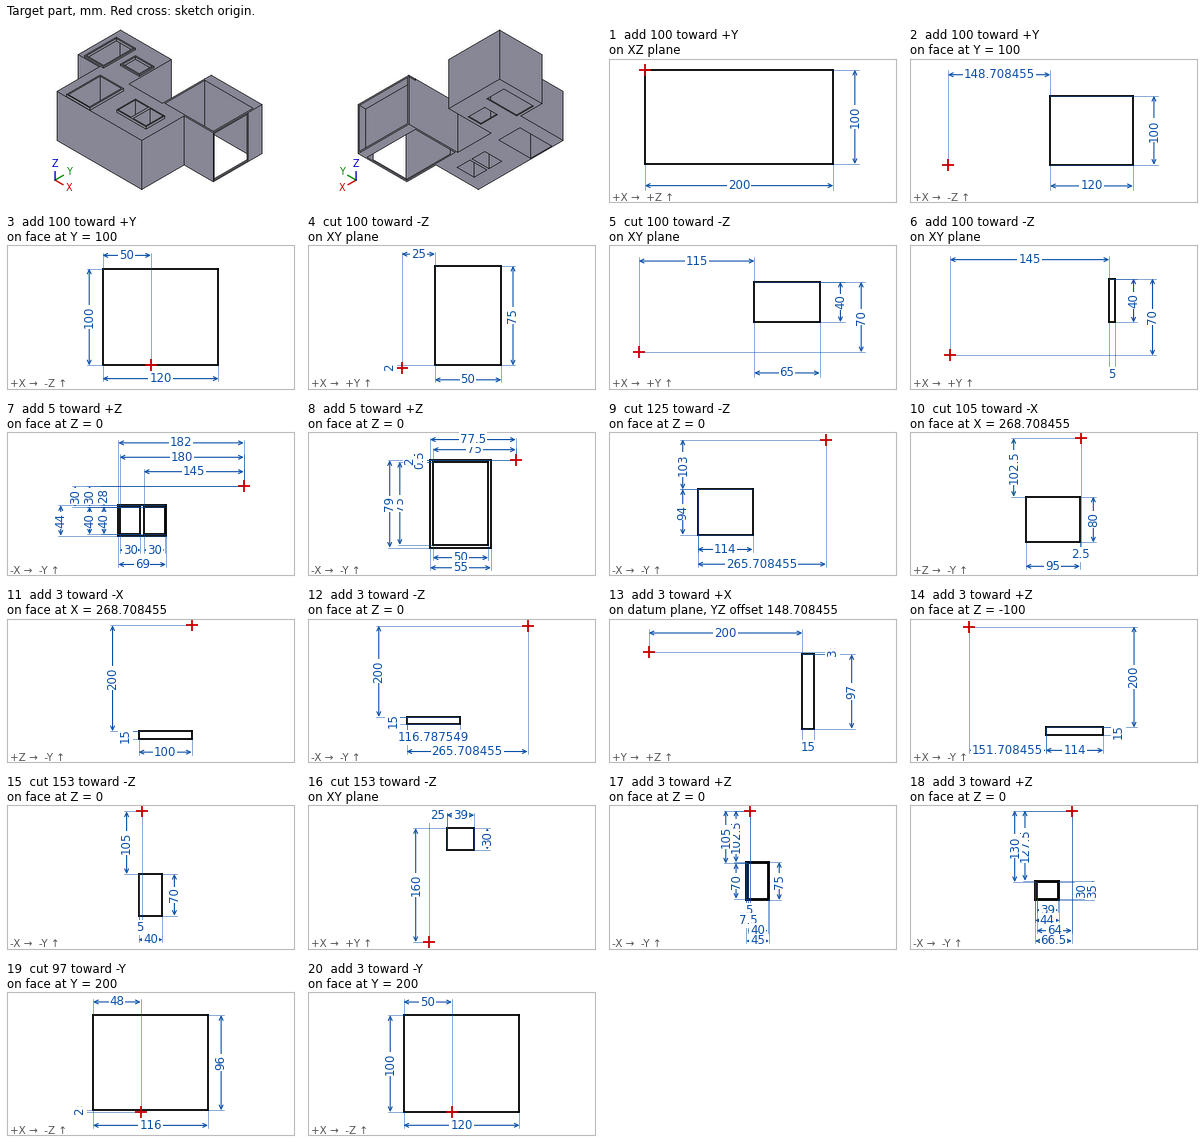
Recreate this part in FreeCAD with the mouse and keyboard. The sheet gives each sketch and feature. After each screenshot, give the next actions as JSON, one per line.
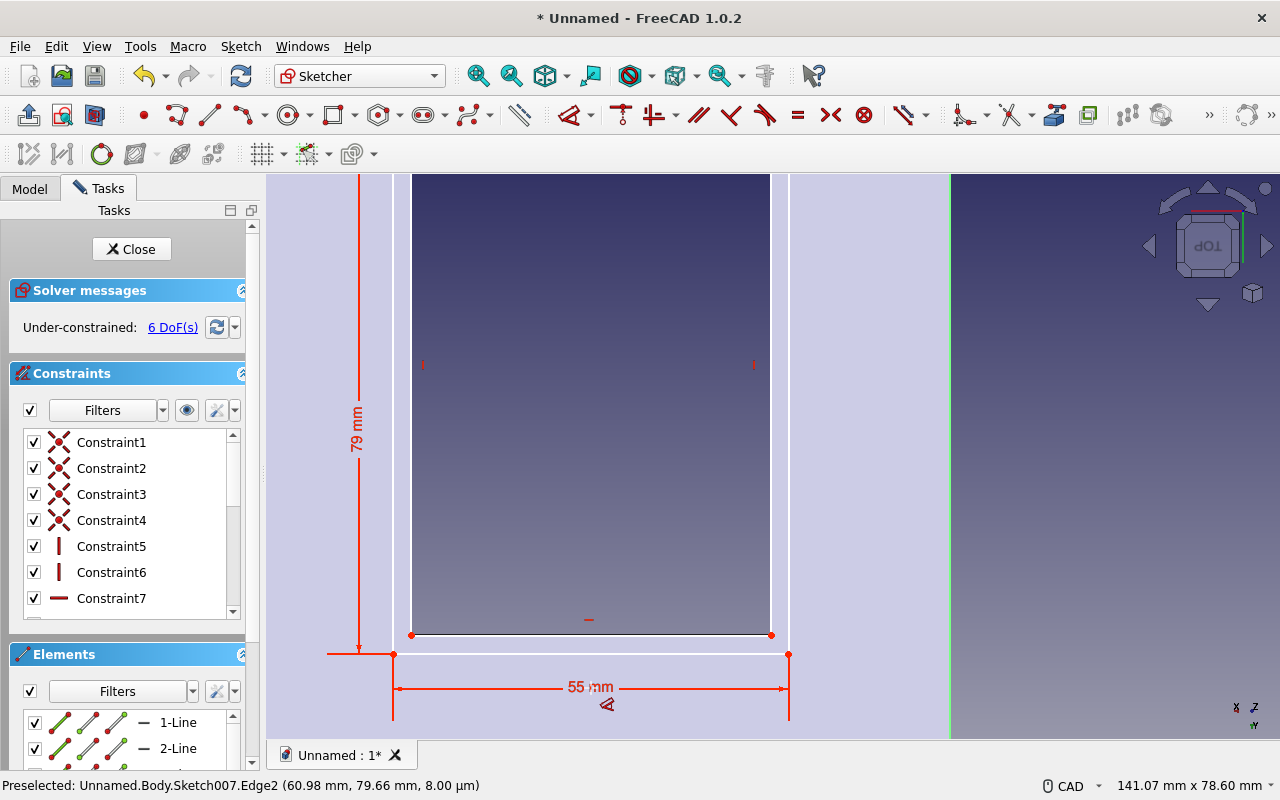
{"action": "left_click", "coordinate": [411, 259]}
{"action": "left_click", "coordinate": [377, 319]}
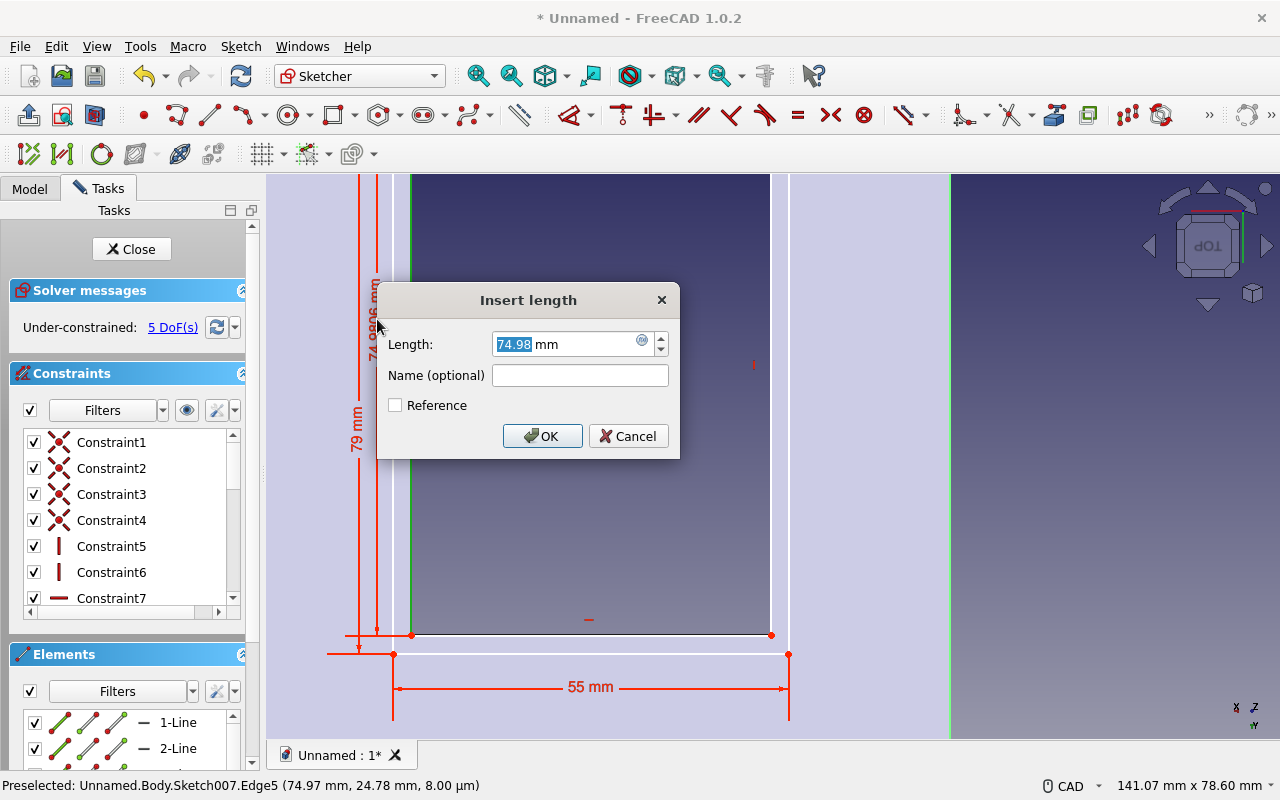
{"action": "type", "text": "75"}
{"action": "key", "text": "Return"}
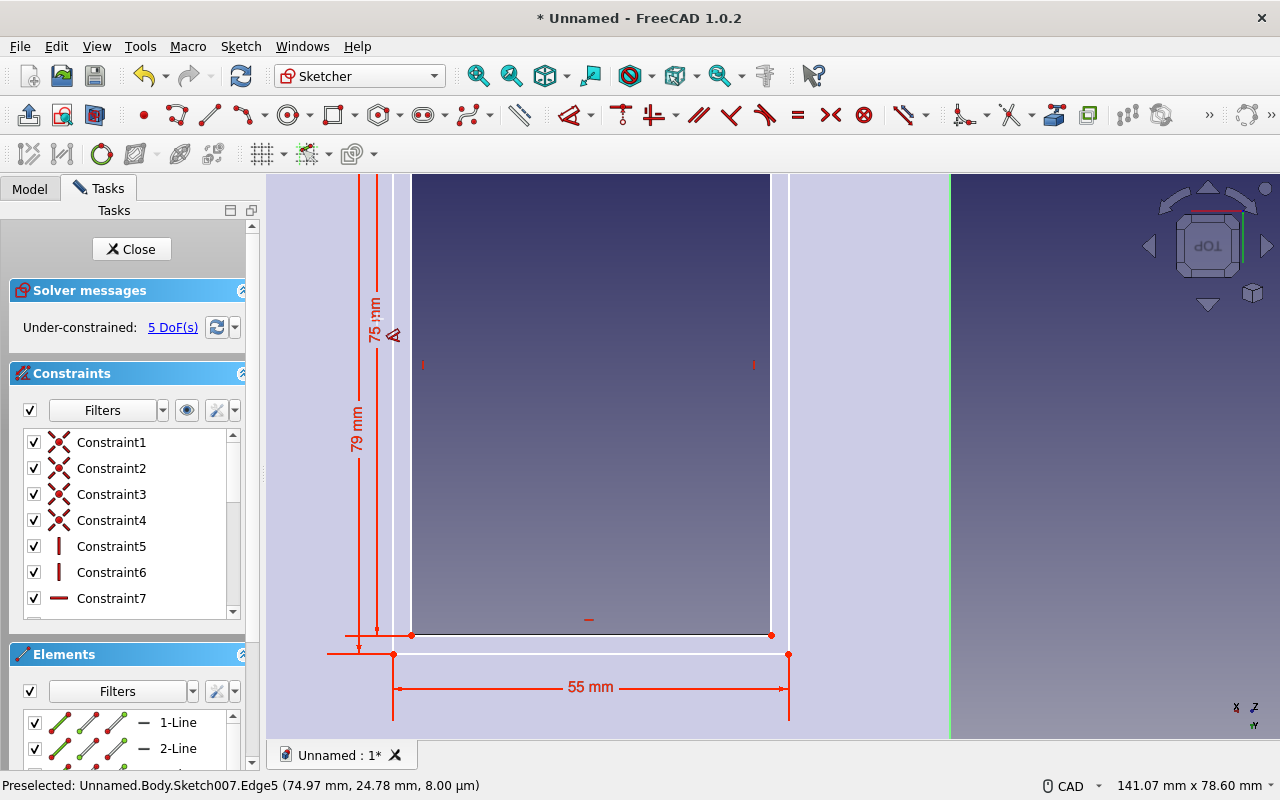
{"action": "left_click", "coordinate": [519, 636]}
{"action": "left_click", "coordinate": [509, 670]}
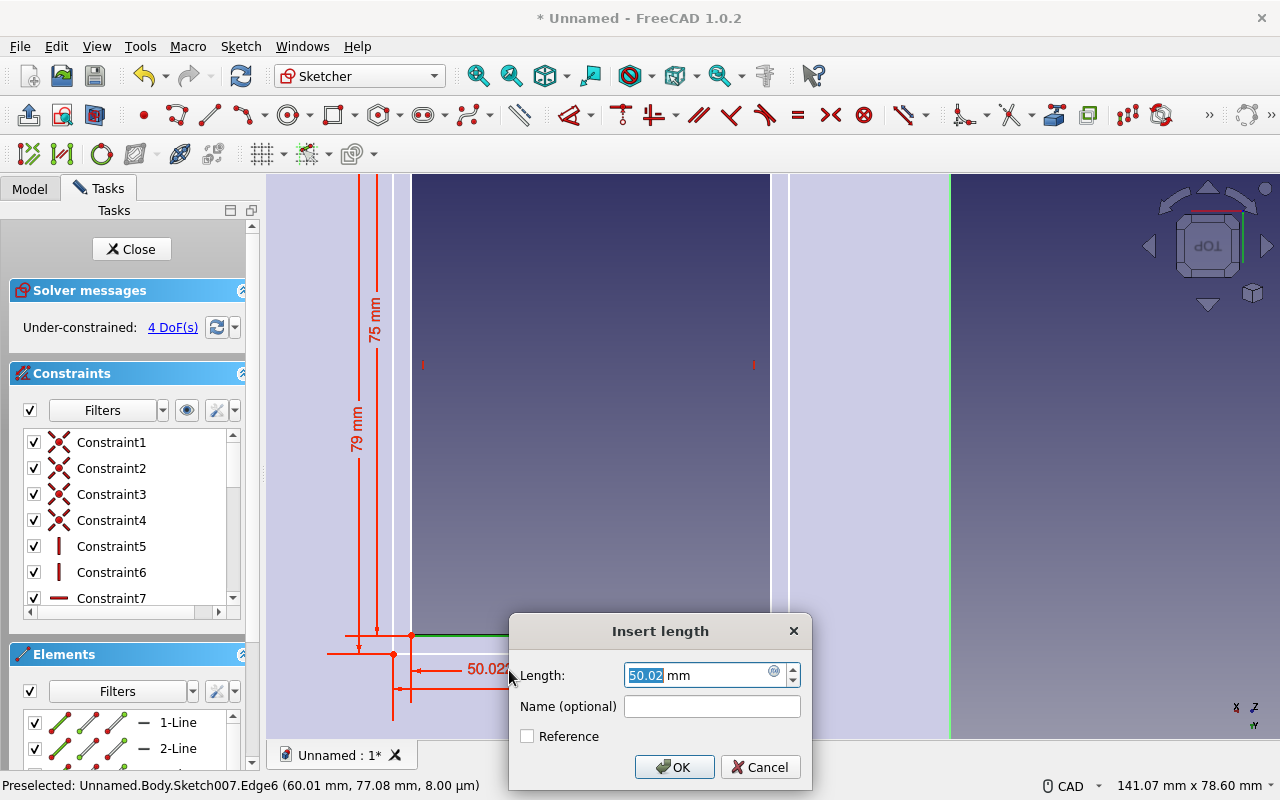
{"action": "type", "text": "50"}
{"action": "key", "text": "Return"}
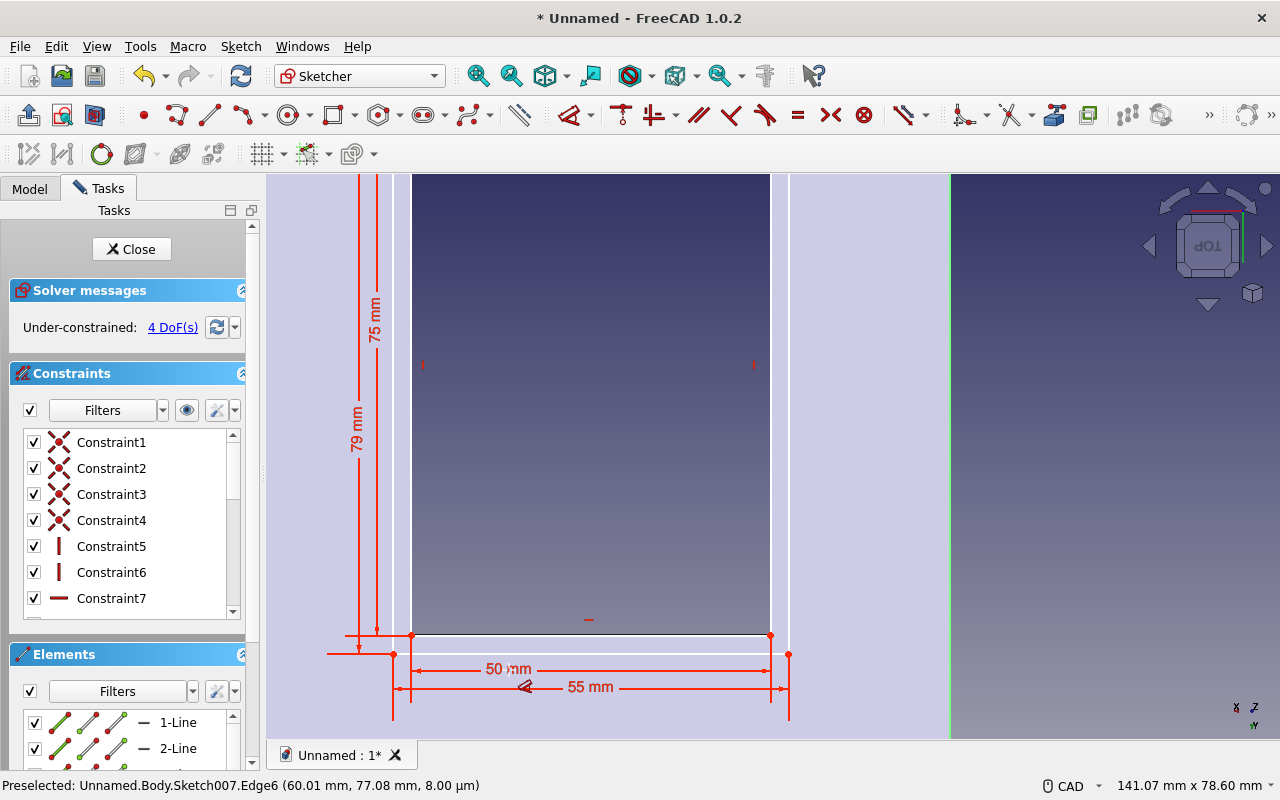
{"action": "scroll", "coordinate": [771, 637], "scroll_direction": "down", "scroll_amount": 2}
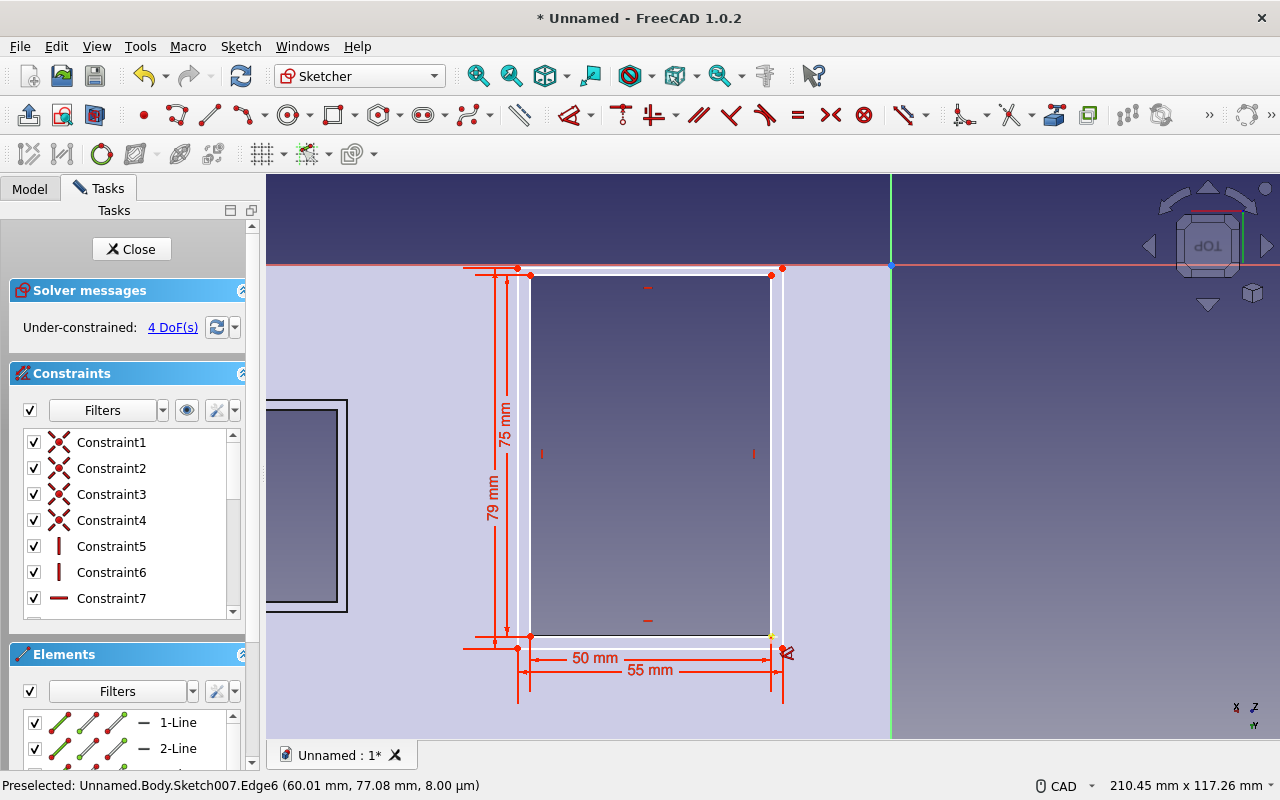
{"action": "scroll", "coordinate": [530, 275], "scroll_direction": "up", "scroll_amount": 8}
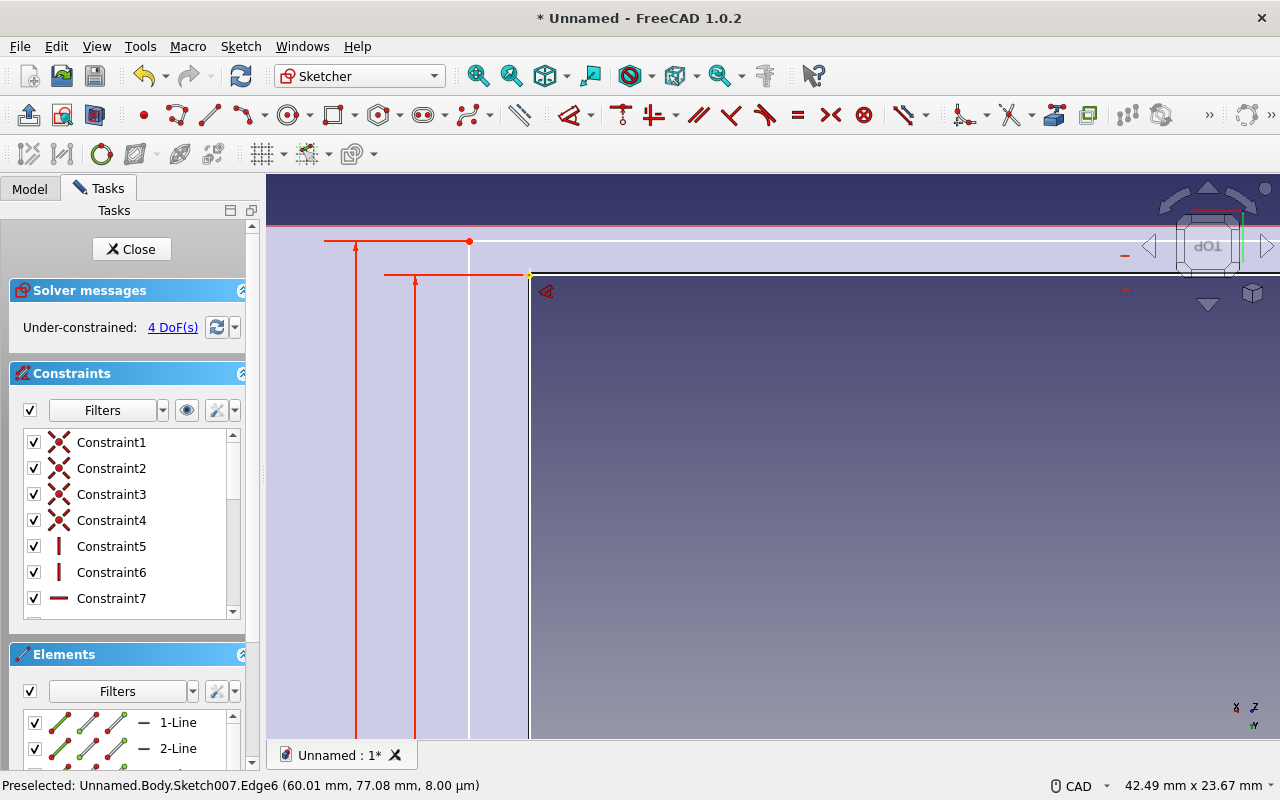
{"action": "left_click", "coordinate": [530, 275]}
{"action": "left_click", "coordinate": [496, 262]}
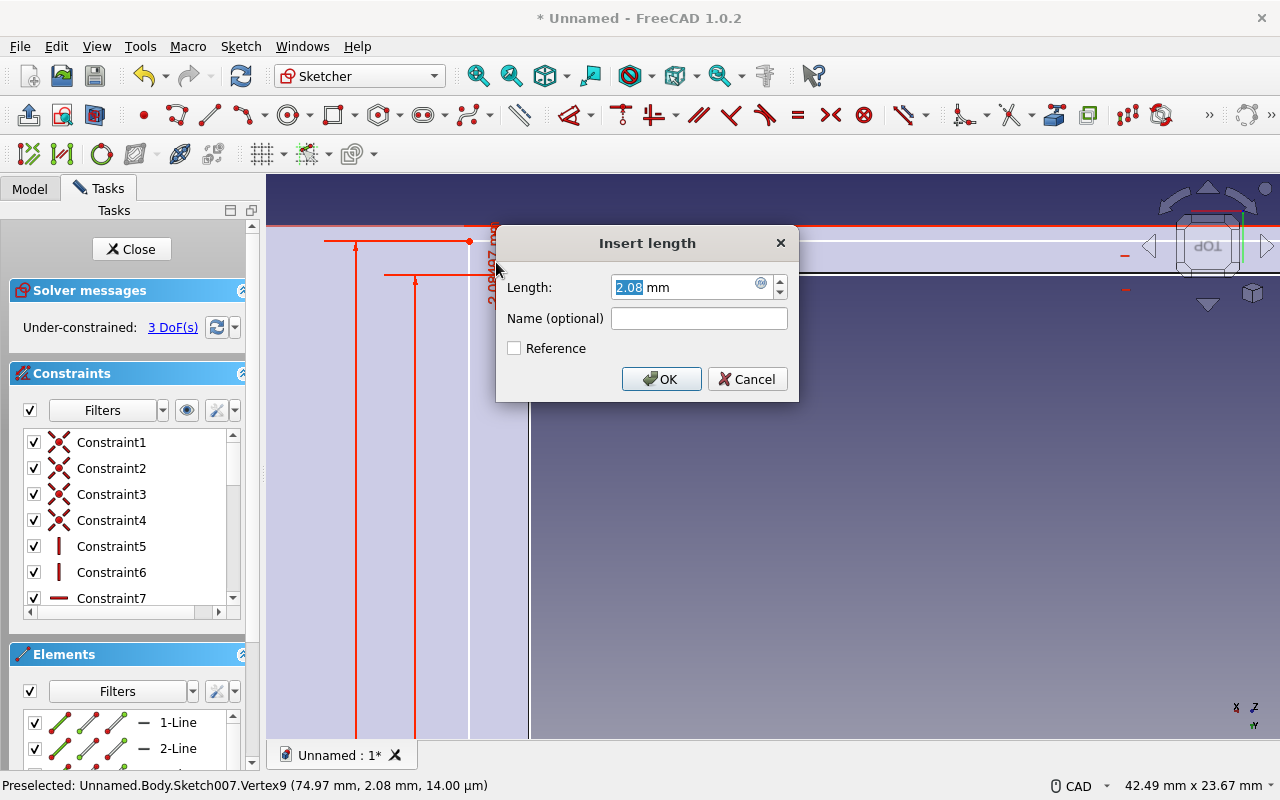
{"action": "type", "text": "2"}
{"action": "key", "text": "Return"}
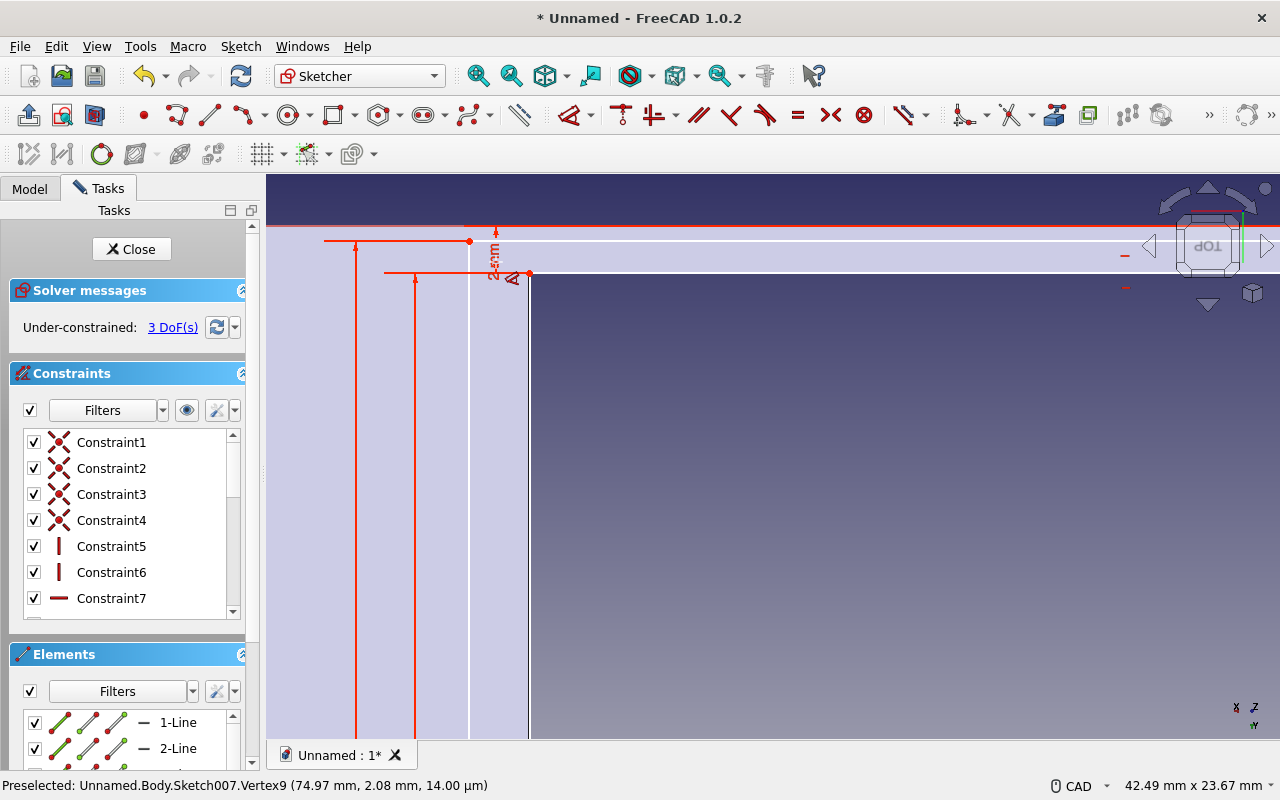
{"action": "scroll", "coordinate": [530, 275], "scroll_direction": "down", "scroll_amount": 8}